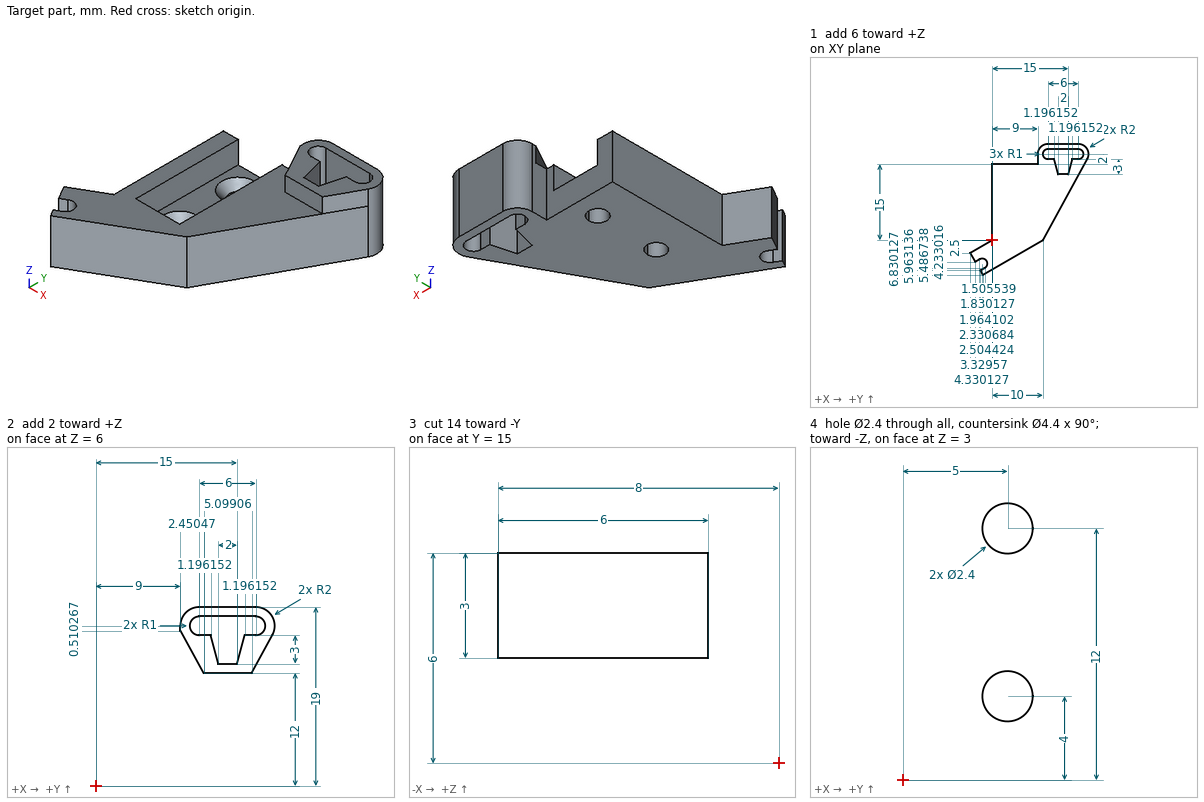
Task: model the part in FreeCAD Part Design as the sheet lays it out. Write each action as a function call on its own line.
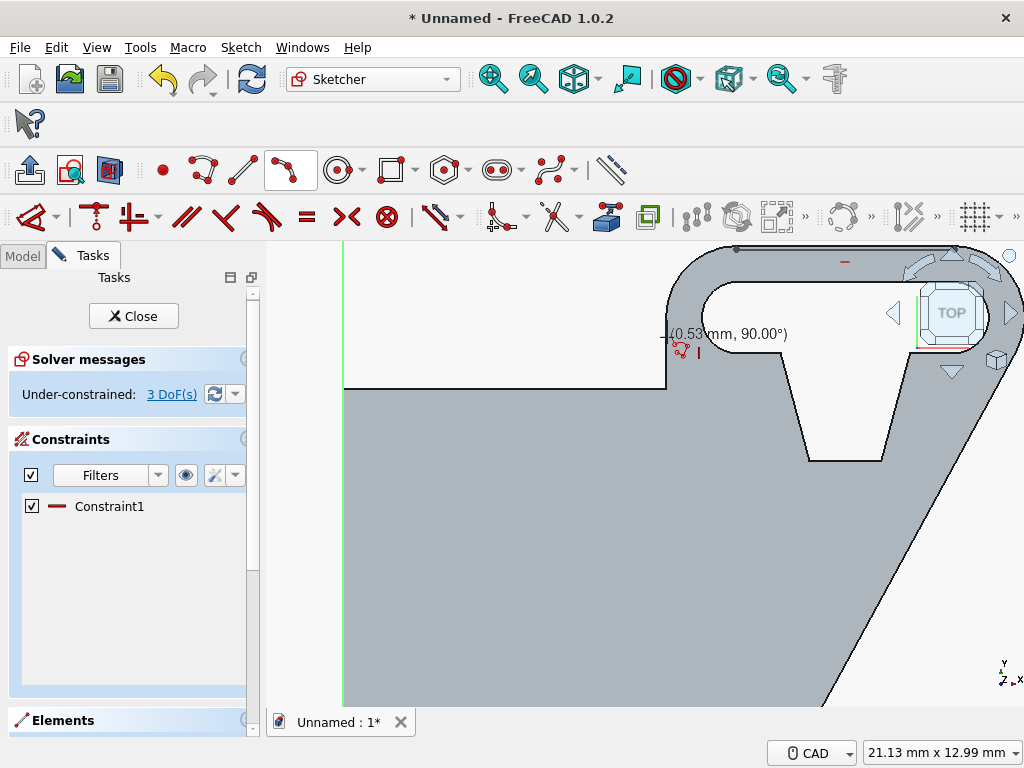
click(666, 336)
click(754, 497)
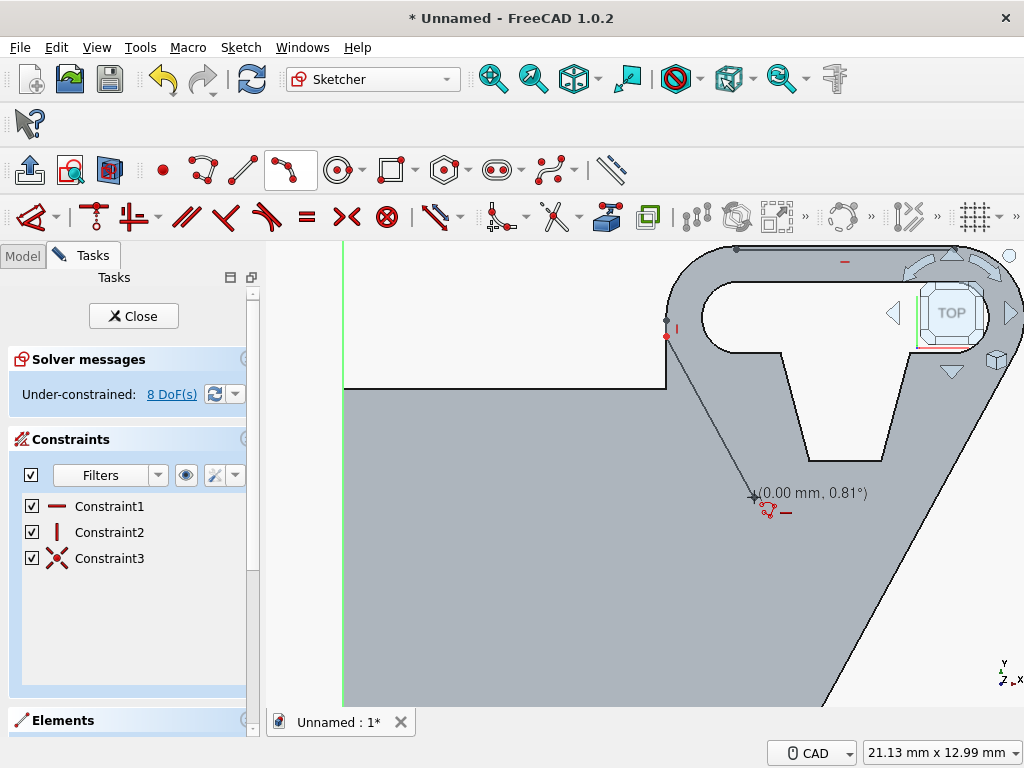
scroll(492, 382, down, 4)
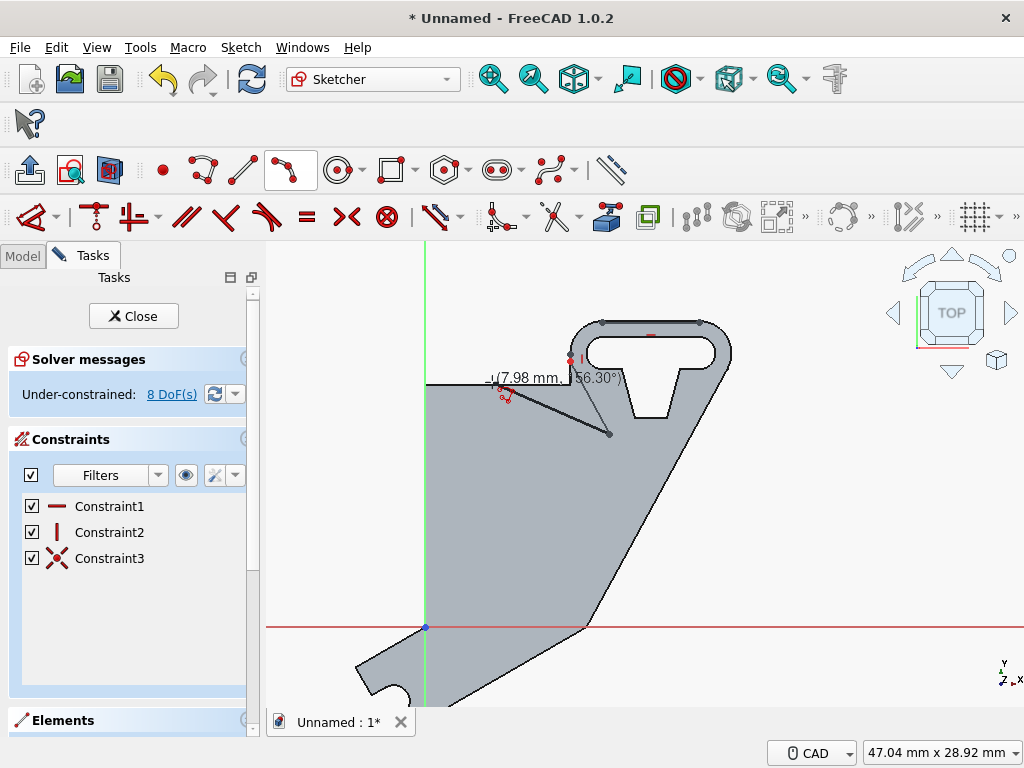
click(692, 434)
click(728, 369)
right_click(728, 369)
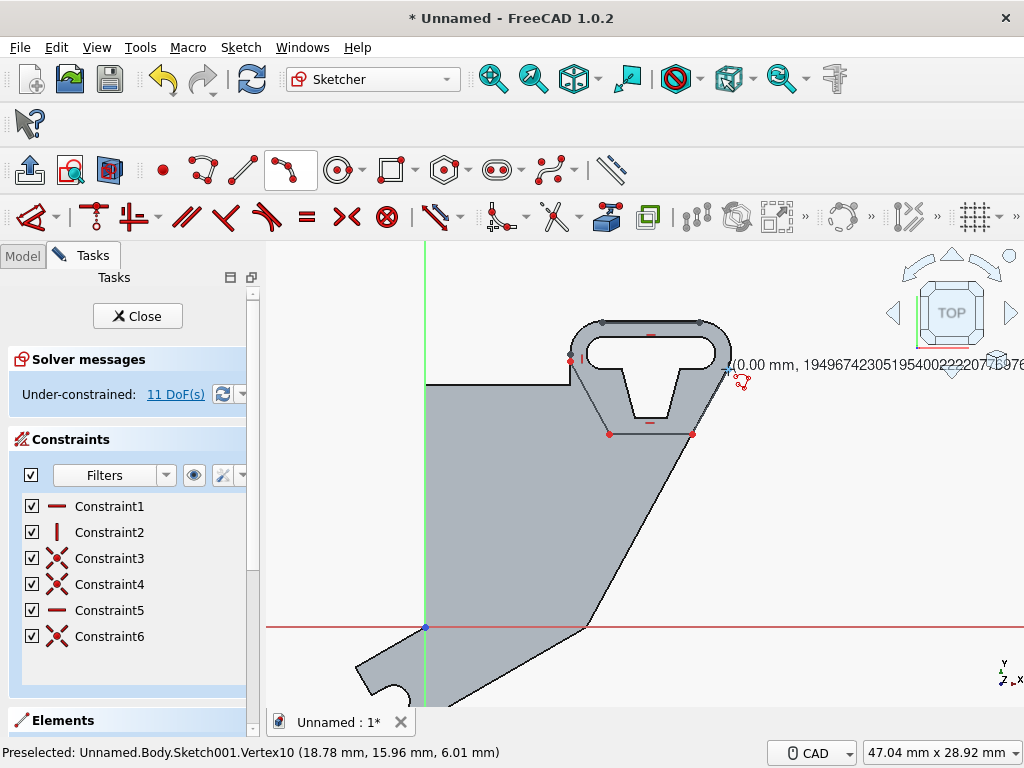
key(g)
key(3)
key(a)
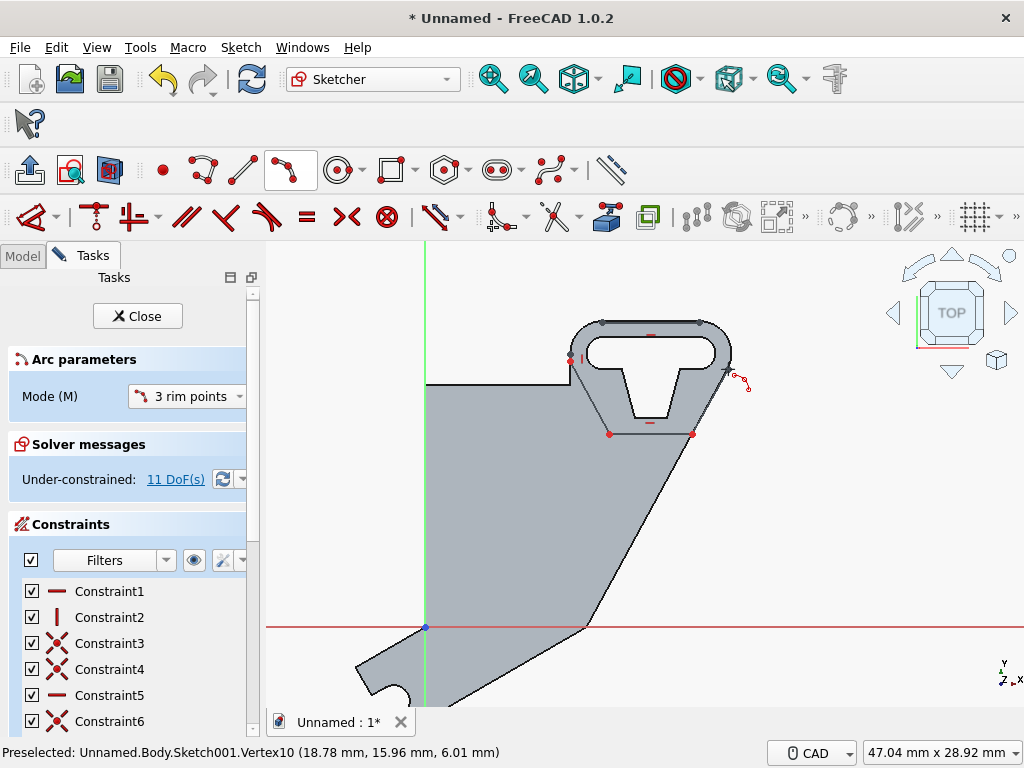
click(602, 323)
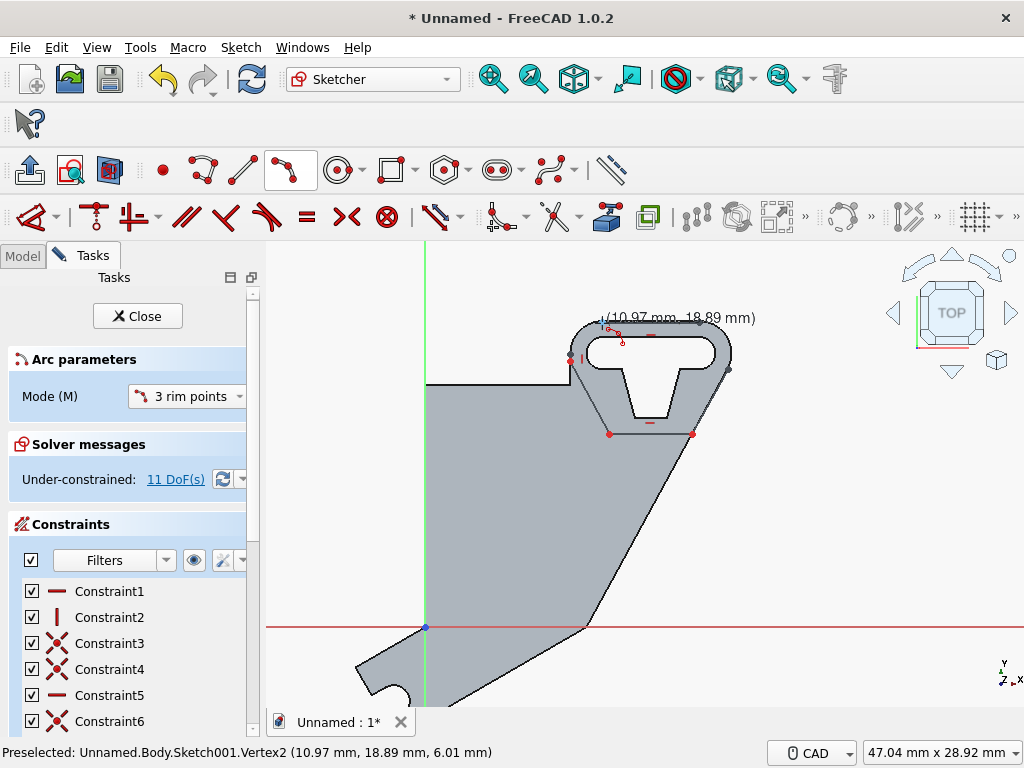
scroll(570, 353, up, 7)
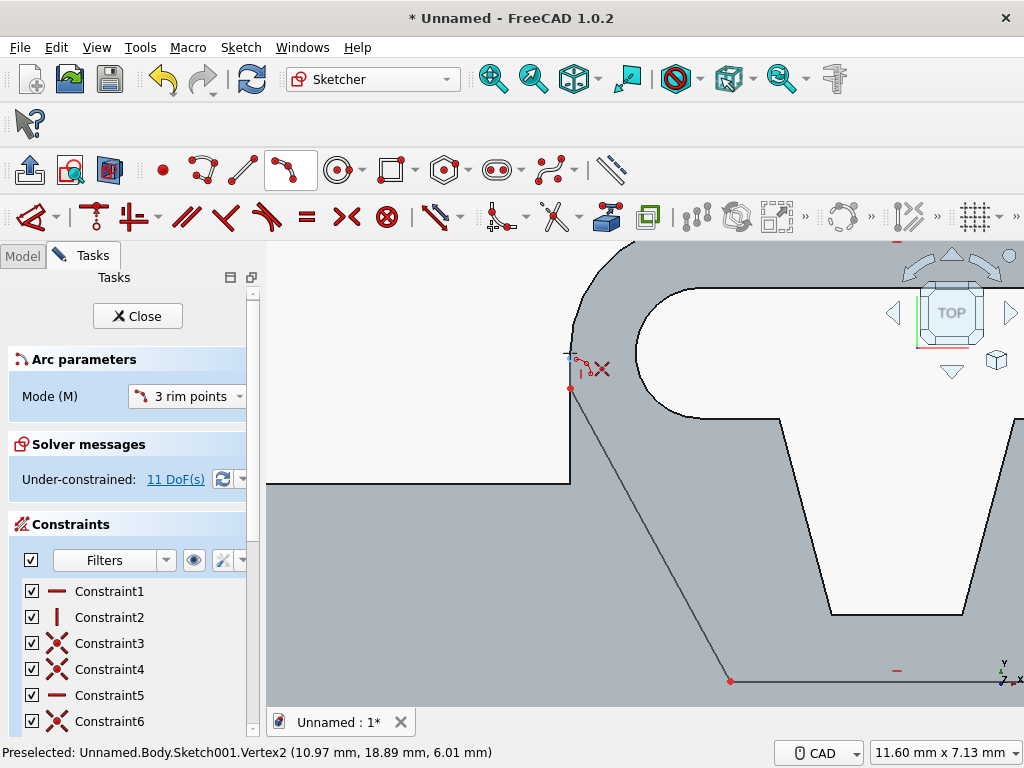
click(570, 358)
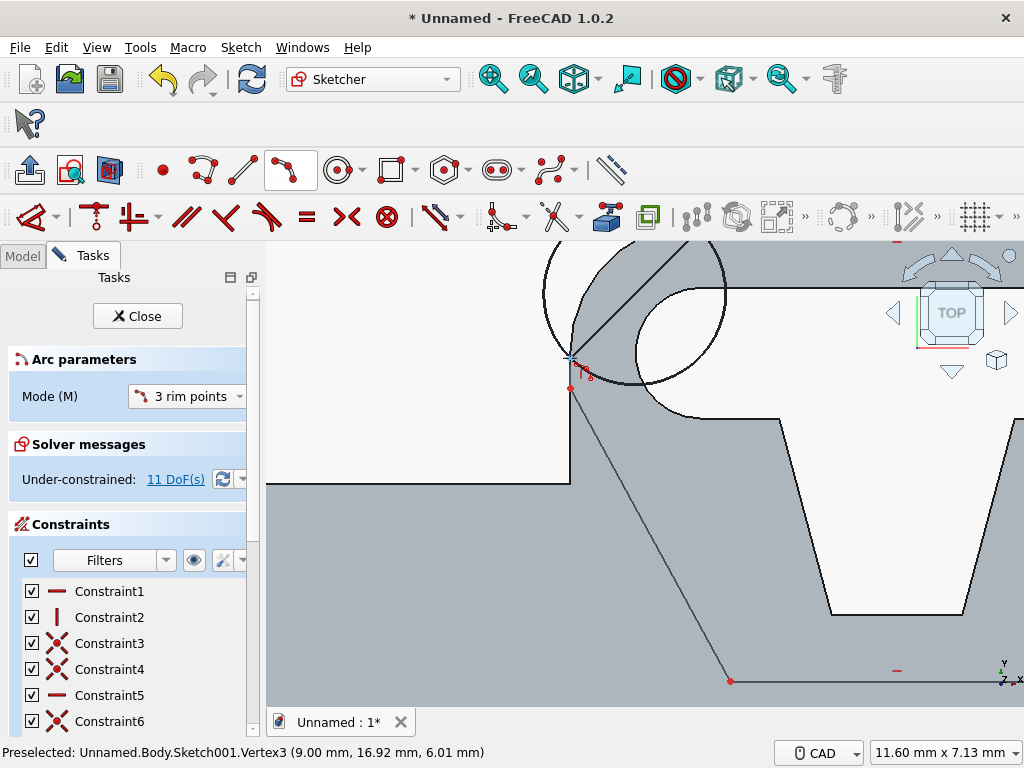
scroll(570, 353, down, 7)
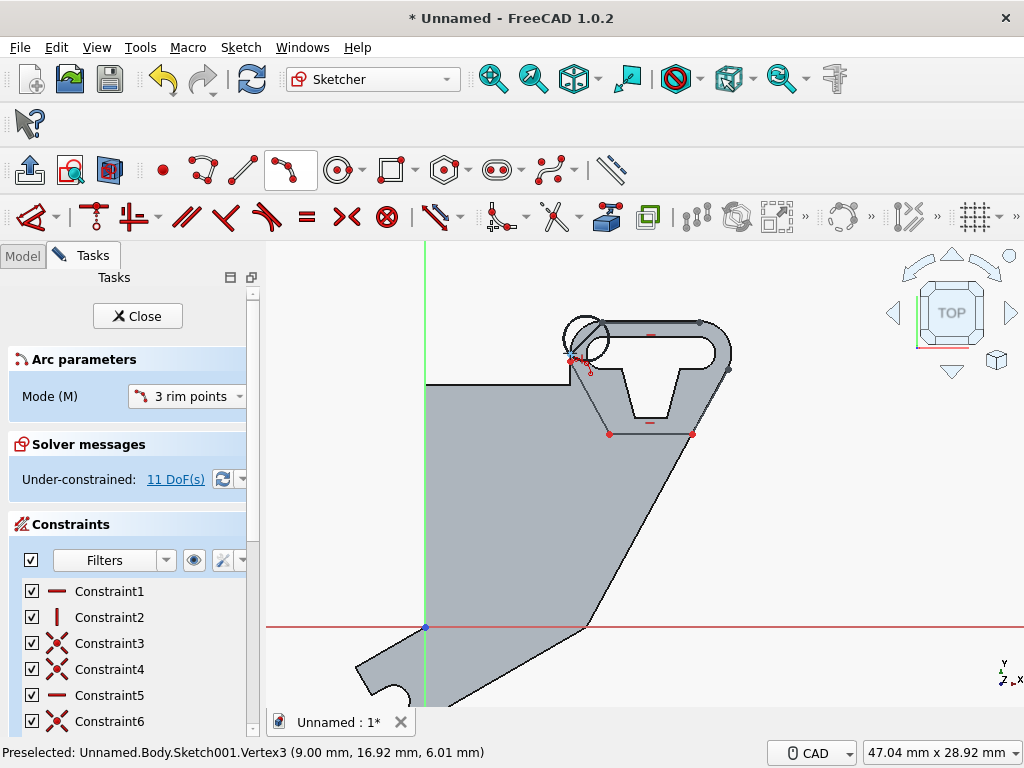
scroll(580, 330, up, 3)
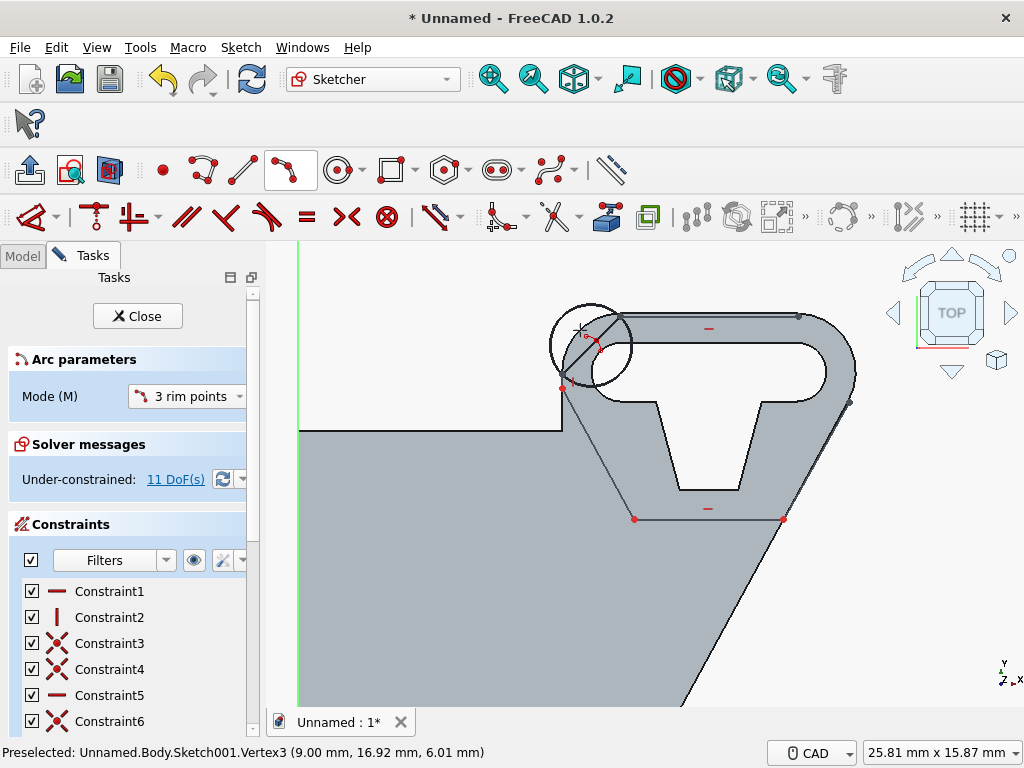
click(579, 331)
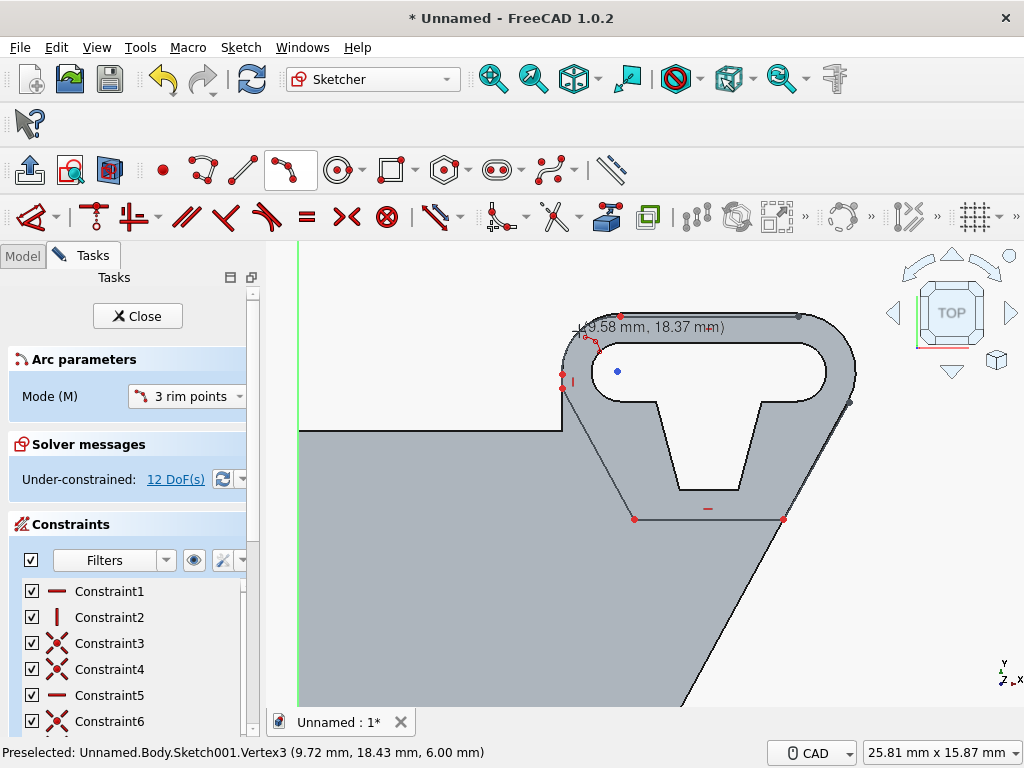
click(849, 403)
click(798, 317)
click(848, 342)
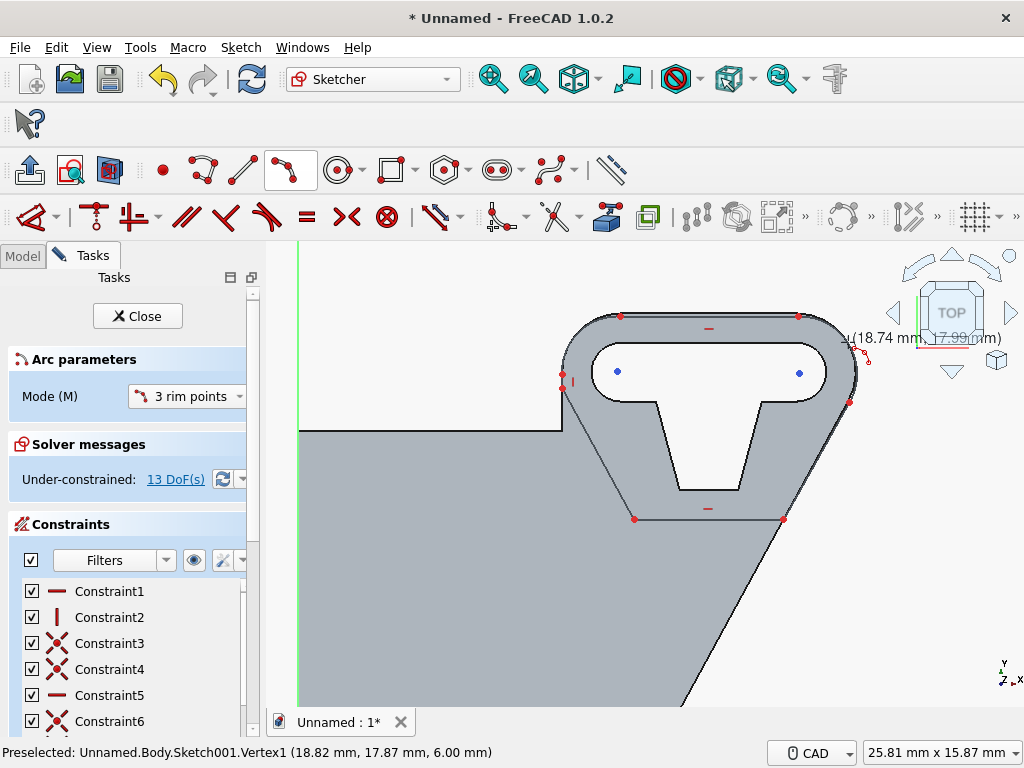
key(g)
key(l)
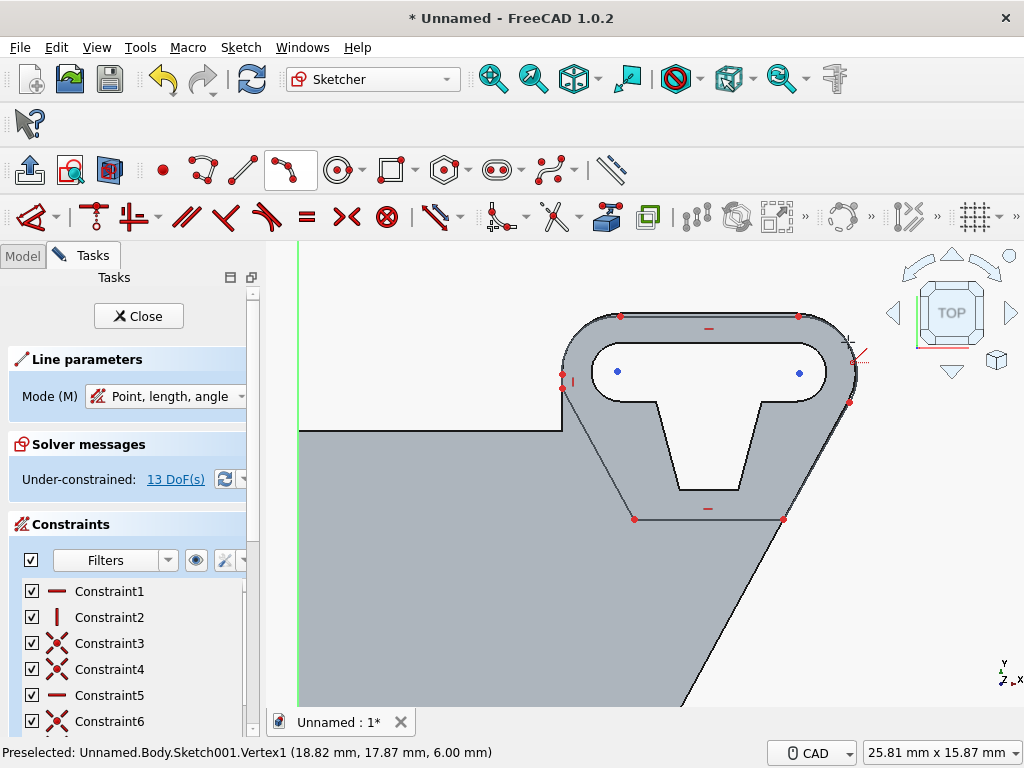
click(621, 343)
click(797, 343)